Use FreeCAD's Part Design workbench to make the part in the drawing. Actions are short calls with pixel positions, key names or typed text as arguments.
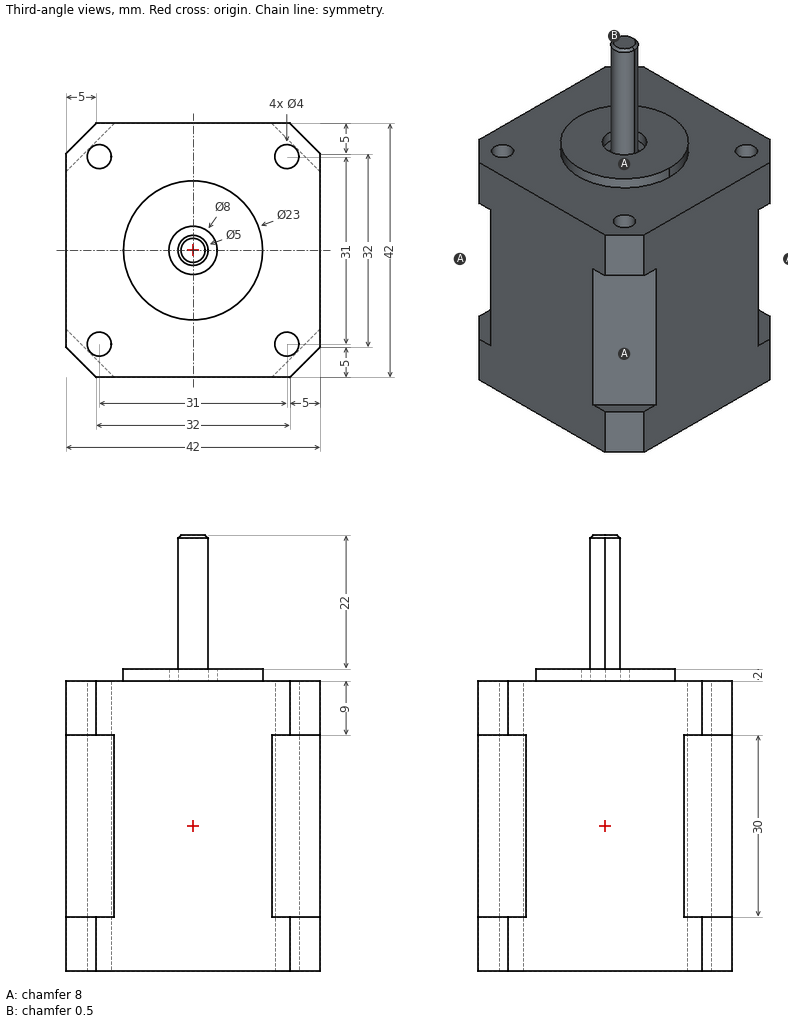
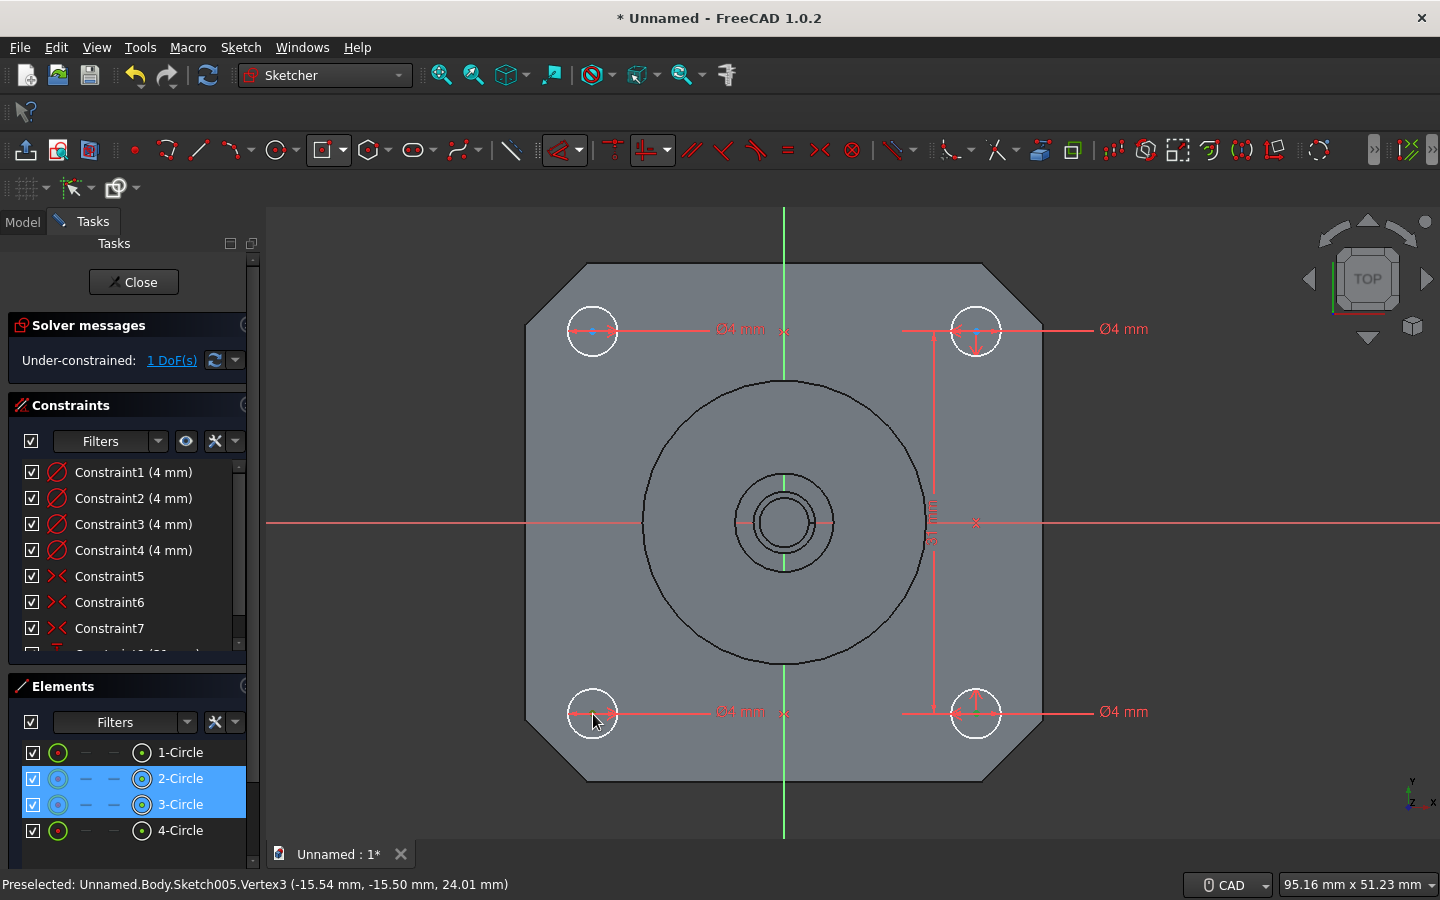
key(l)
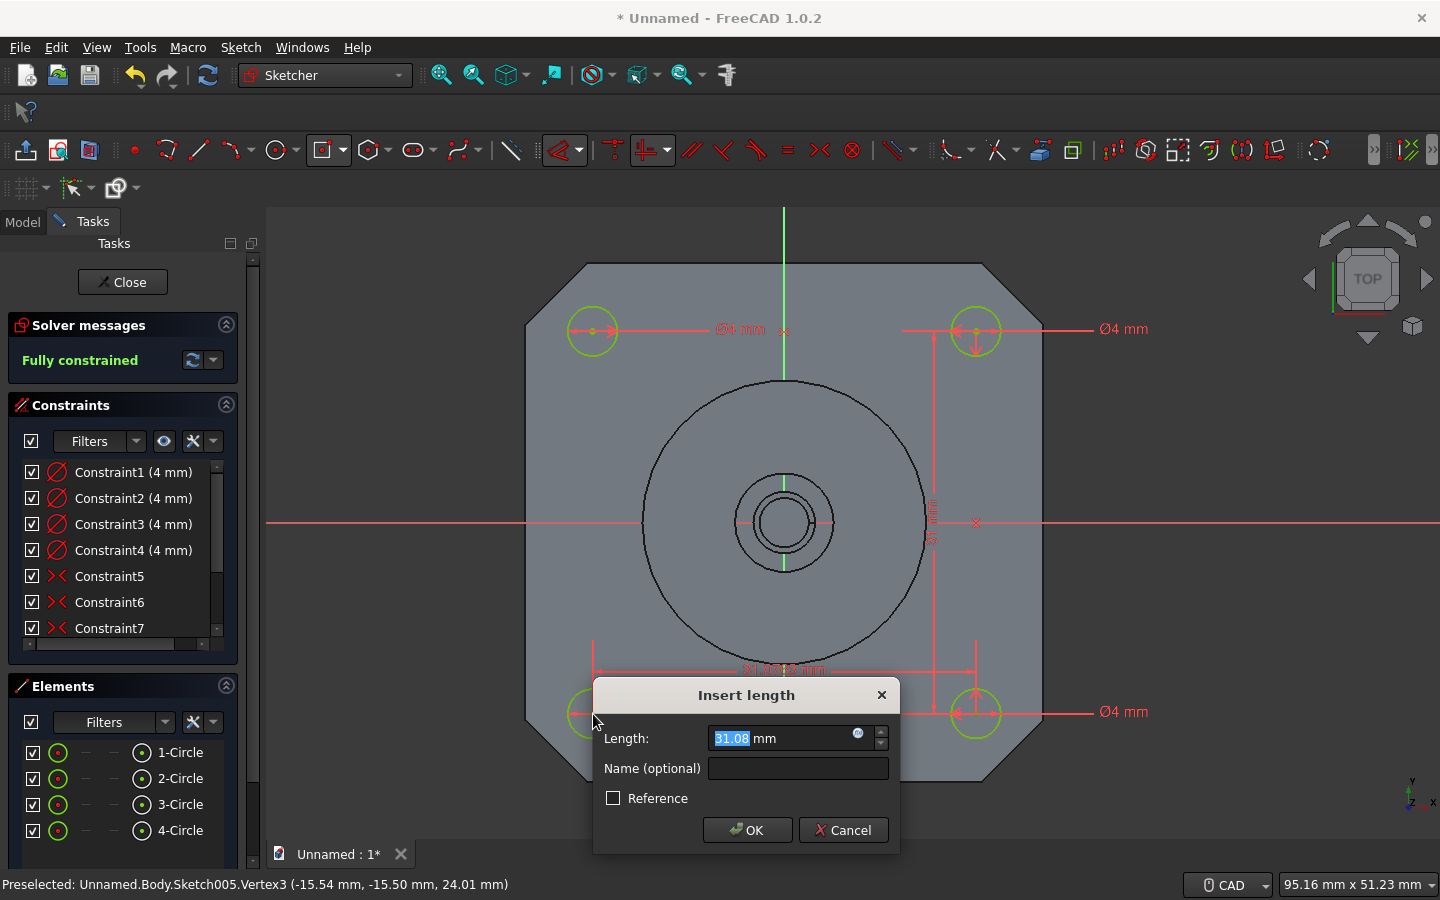
text(31)
key(Return)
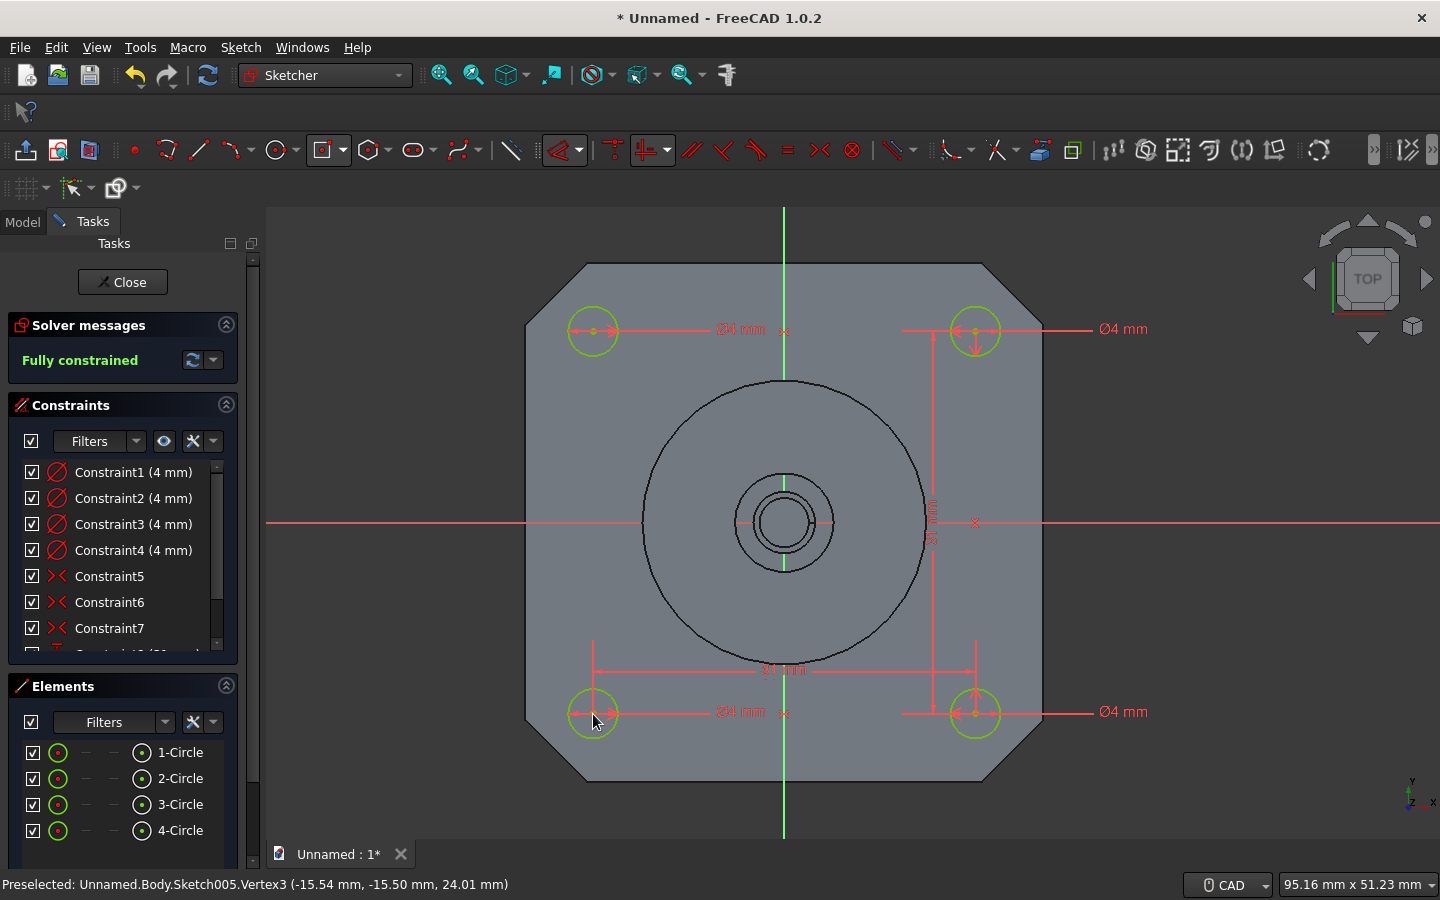
click(123, 282)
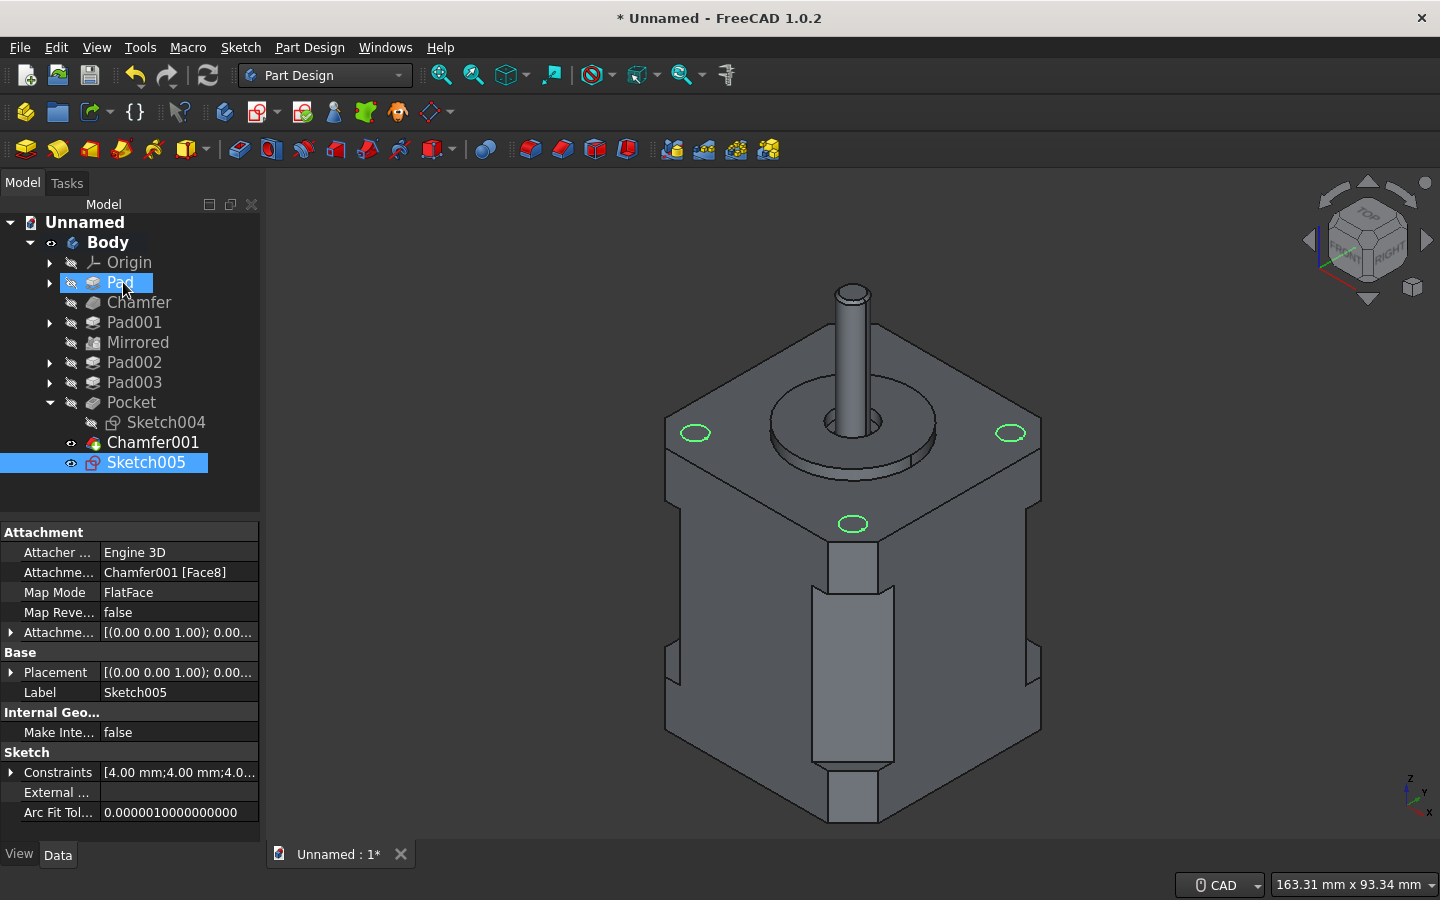
click(240, 150)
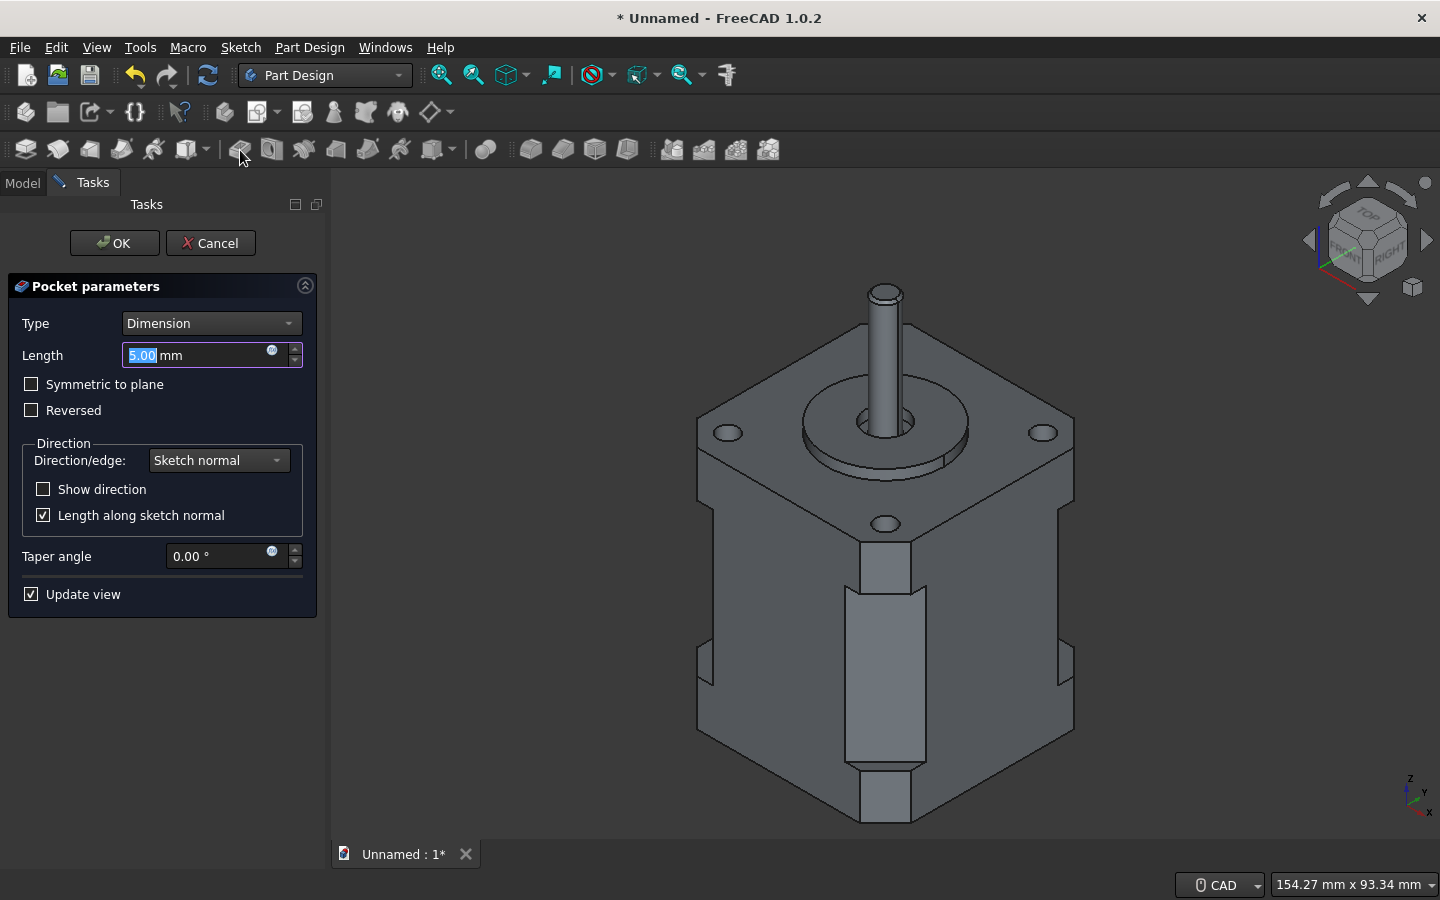
click(212, 324)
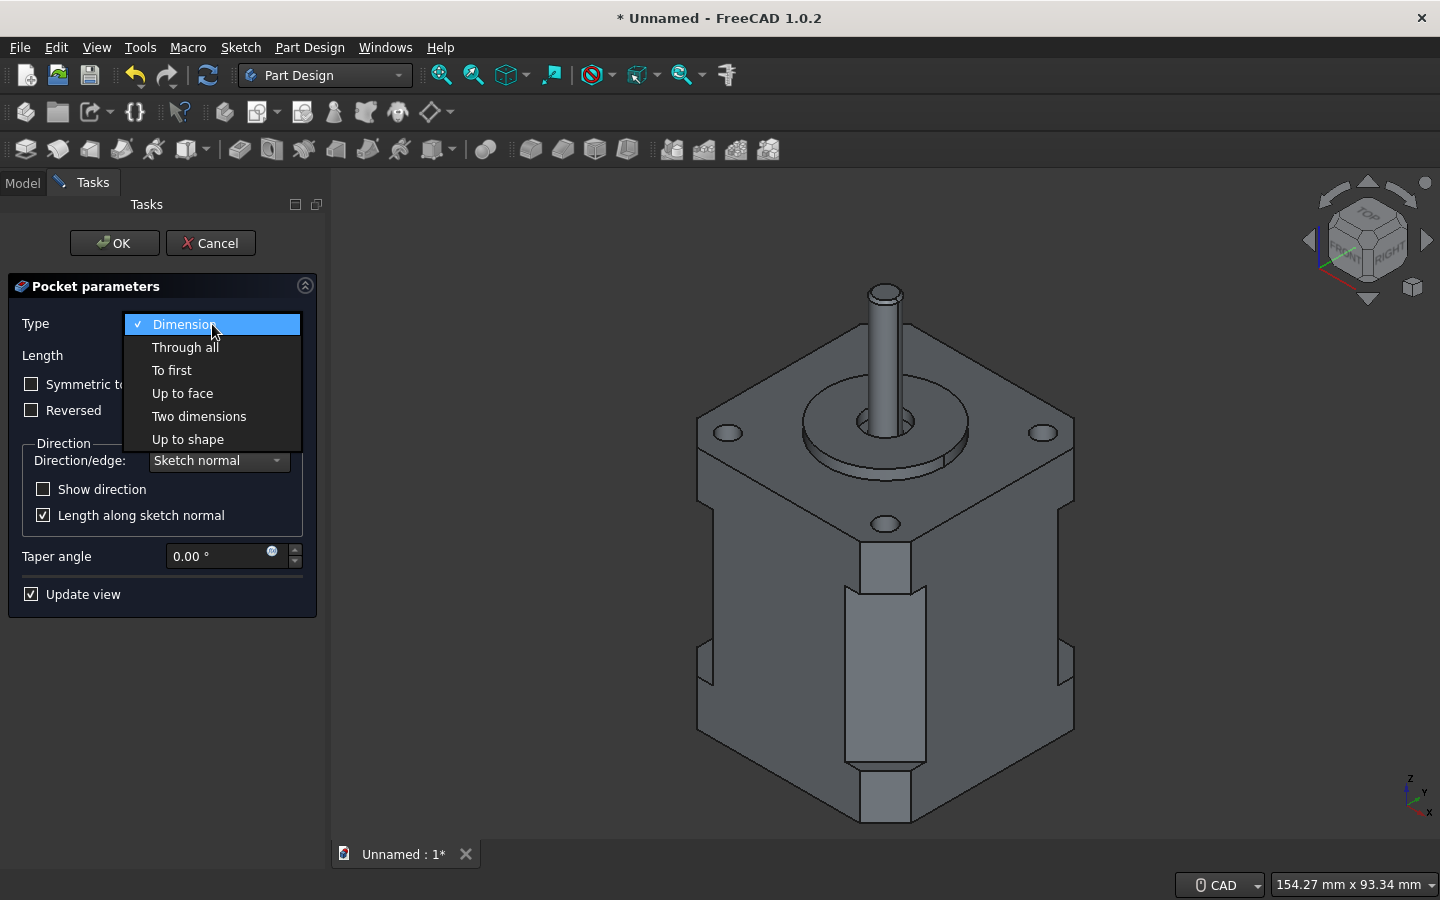
click(212, 348)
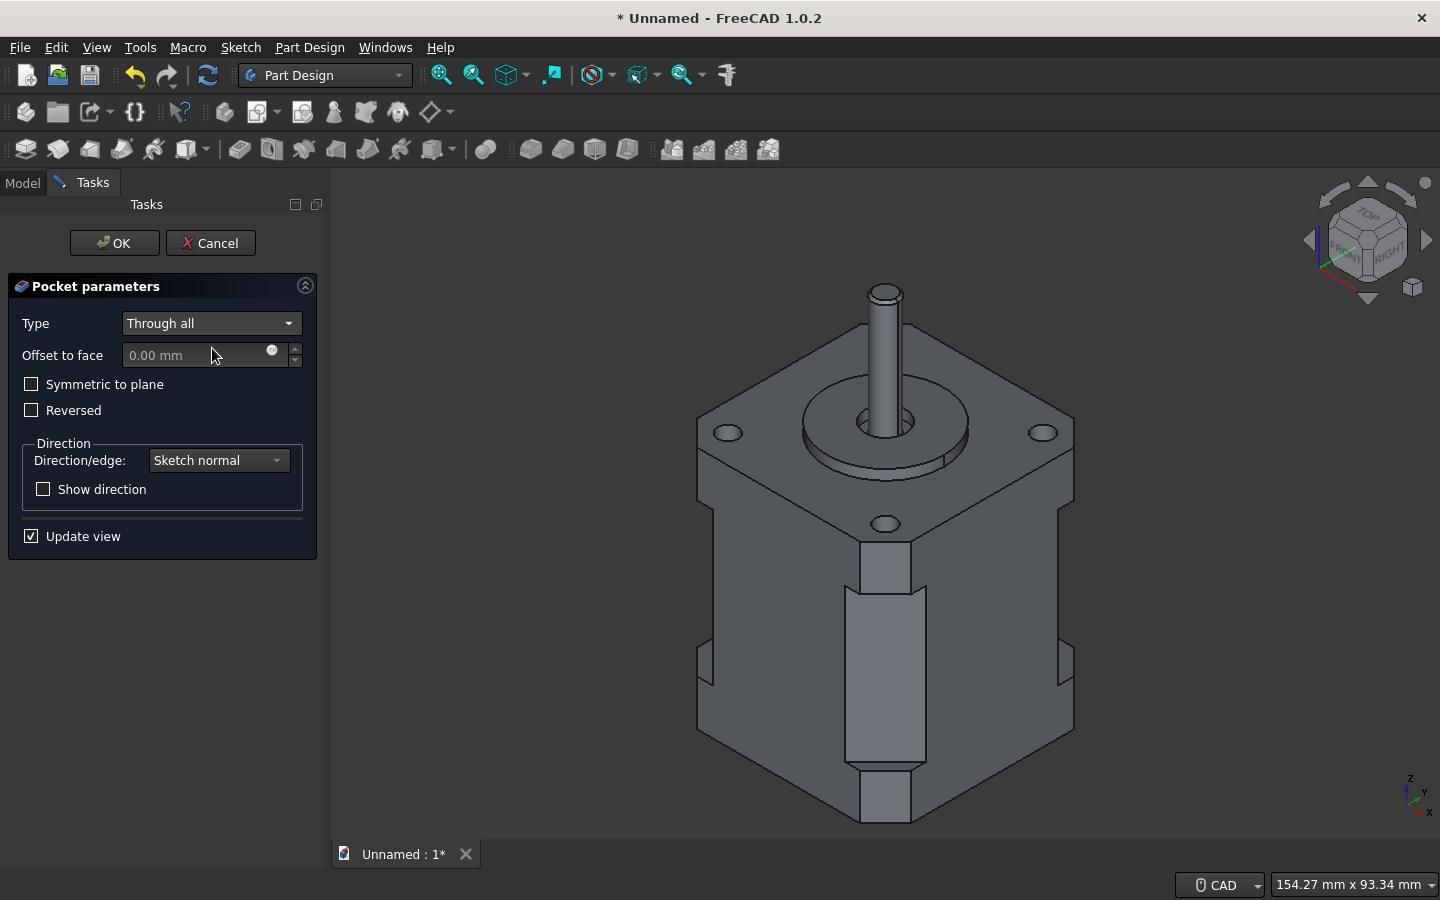
click(115, 243)